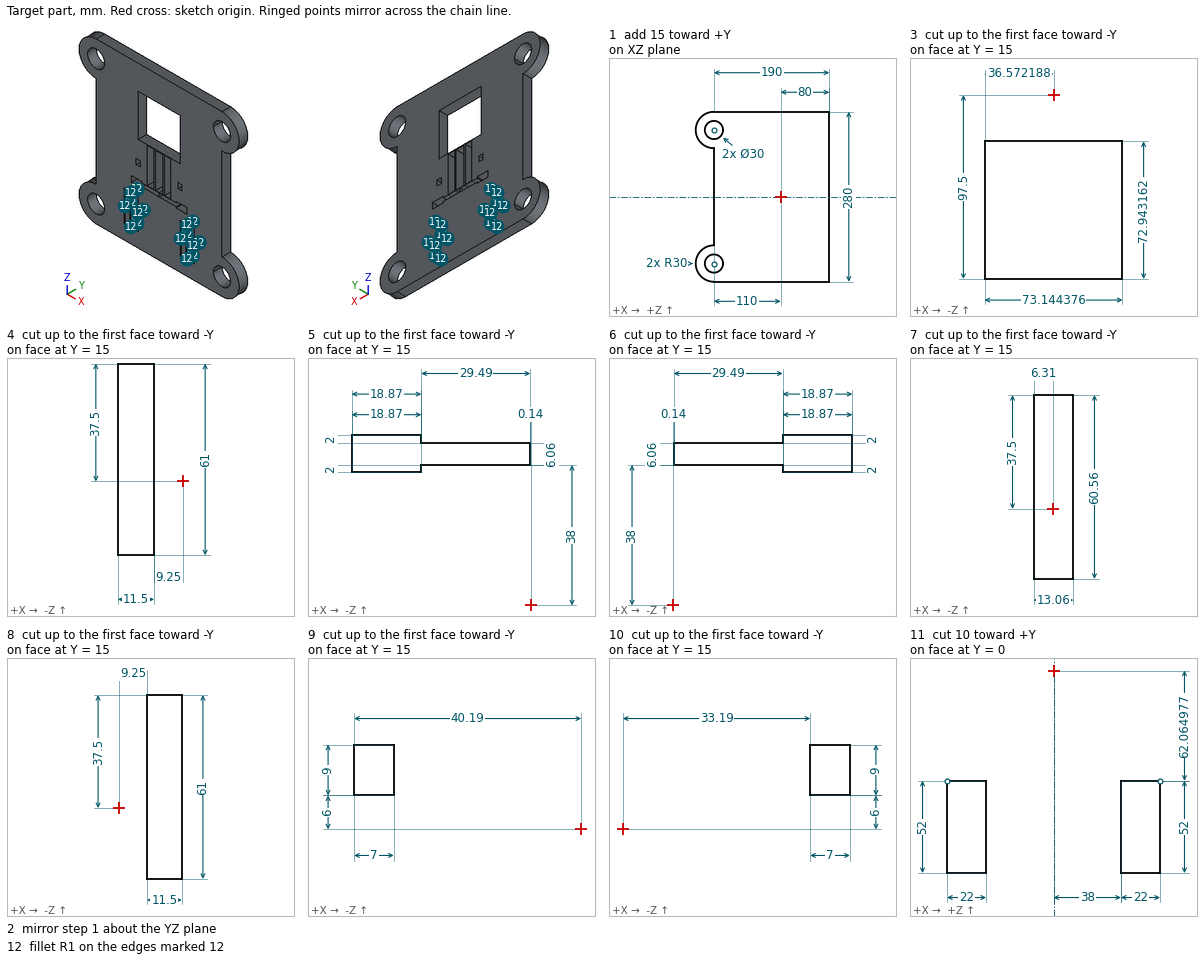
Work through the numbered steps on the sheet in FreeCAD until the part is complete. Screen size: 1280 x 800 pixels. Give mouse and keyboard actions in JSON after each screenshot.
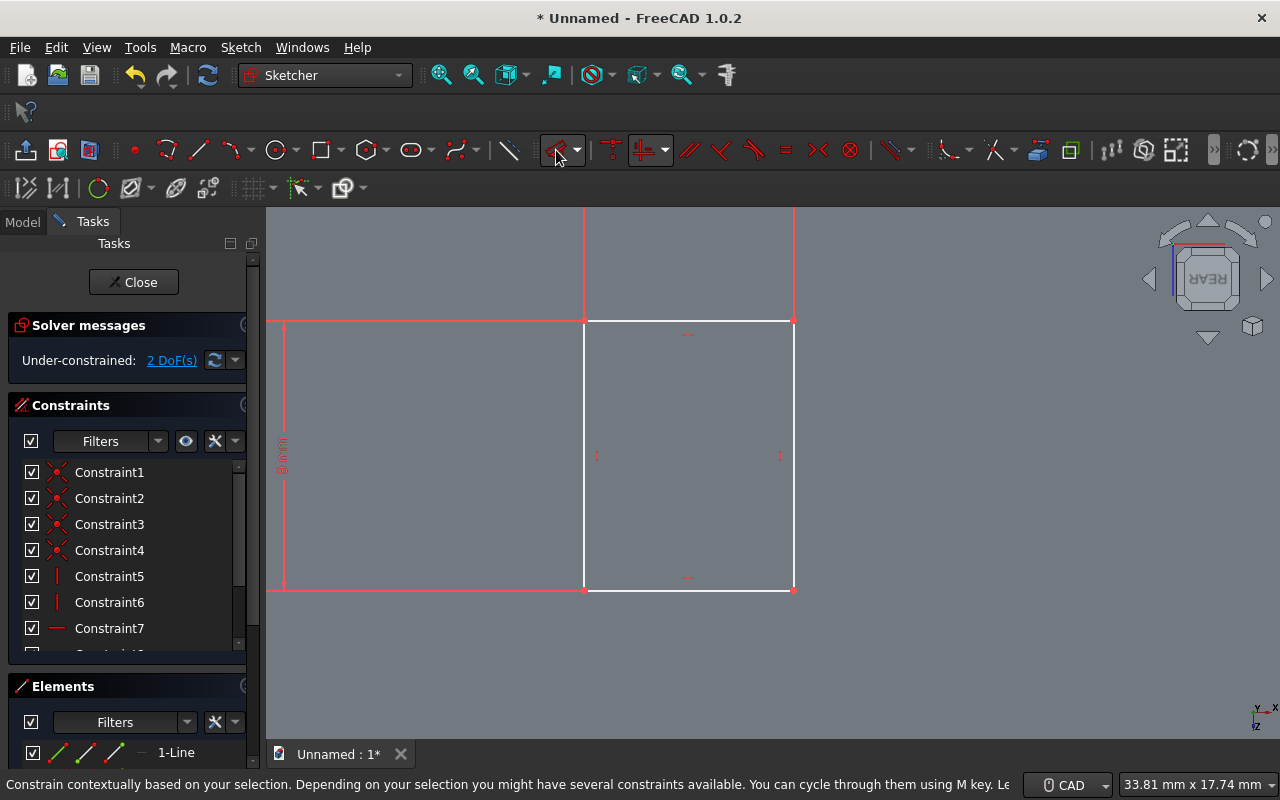
{"action": "left_click", "coordinate": [584, 591]}
{"action": "left_click", "coordinate": [618, 651]}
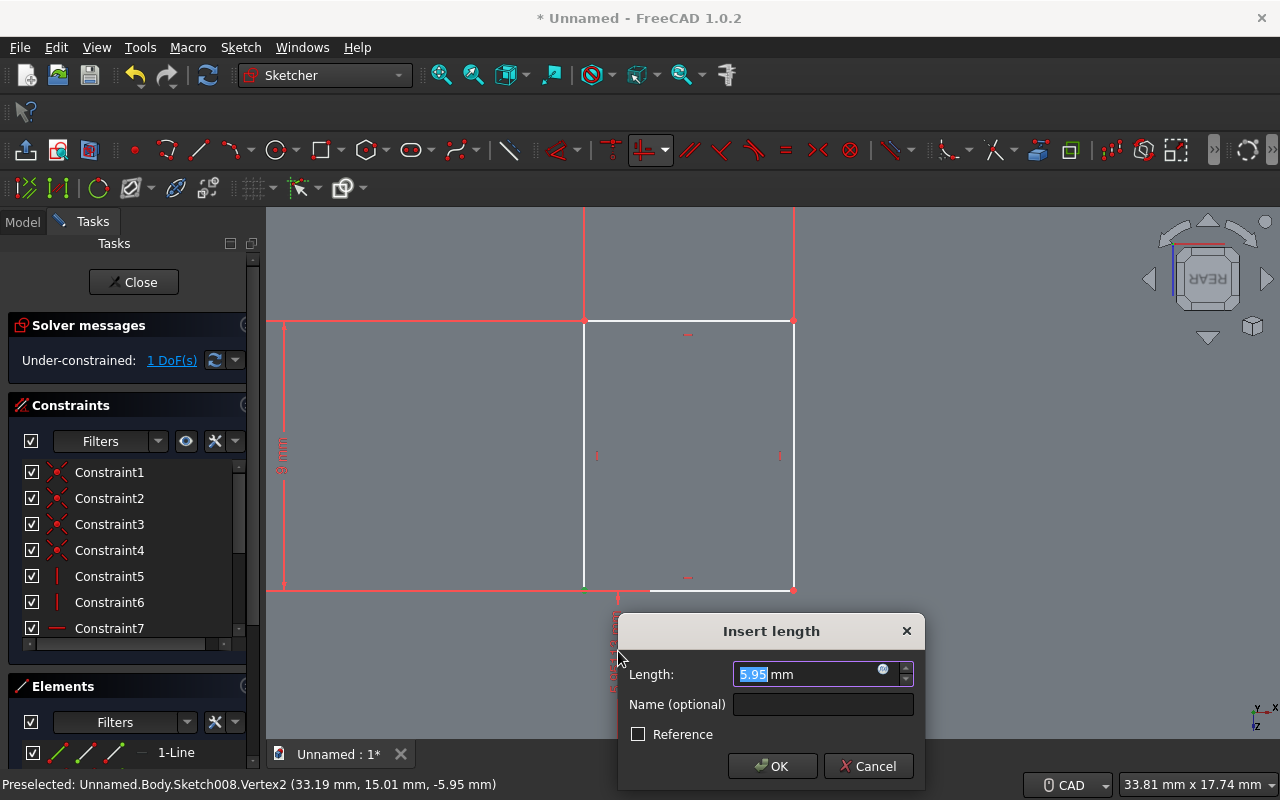
{"action": "type", "text": "6"}
{"action": "key", "text": "Return"}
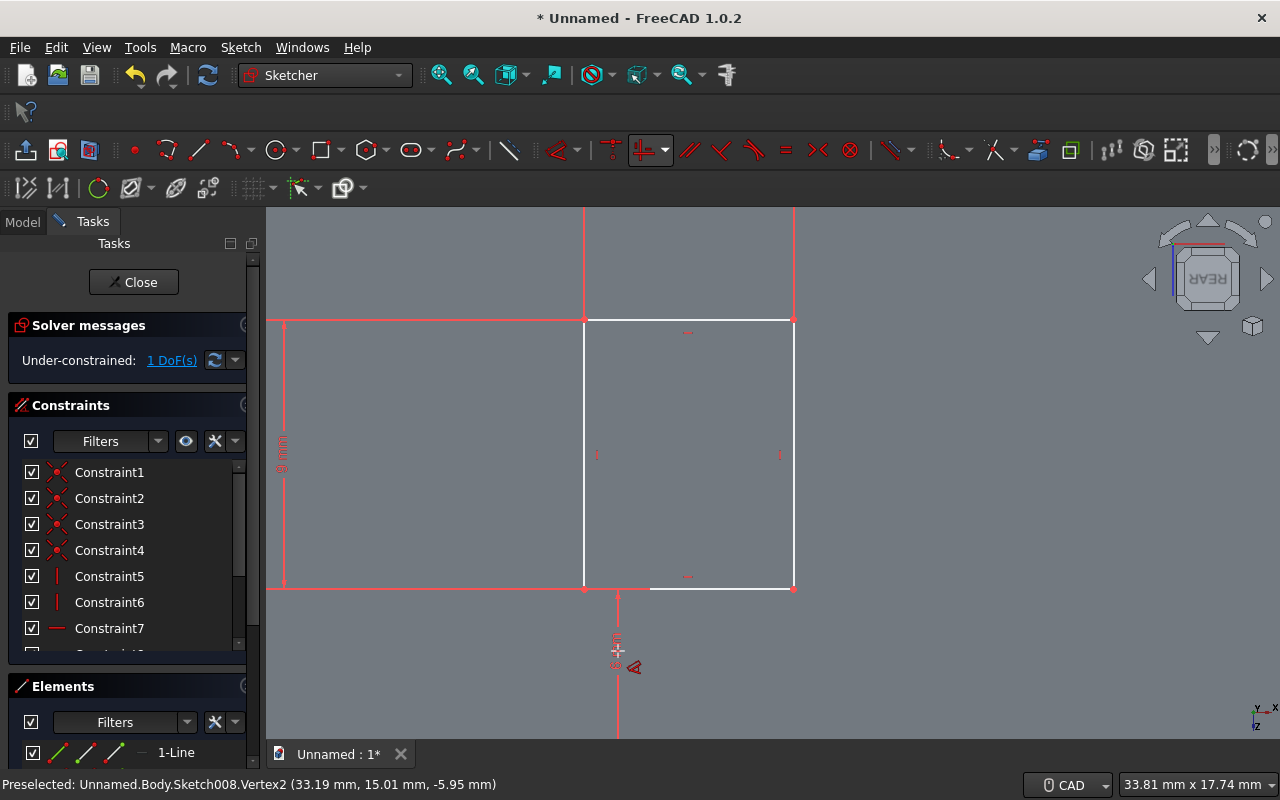
{"action": "left_click", "coordinate": [584, 320]}
{"action": "left_click", "coordinate": [439, 286]}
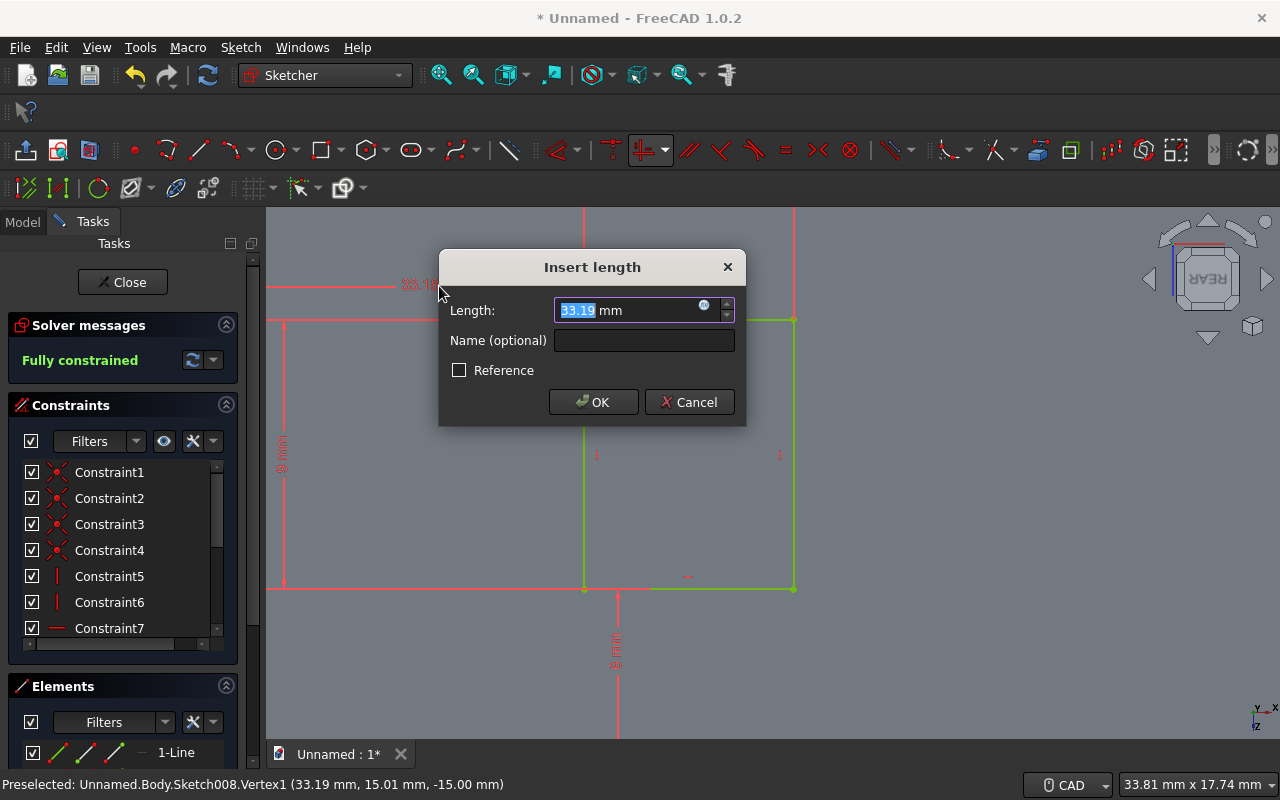
{"action": "type", "text": "33.19"}
{"action": "key", "text": "Return"}
{"action": "key", "text": "Escape"}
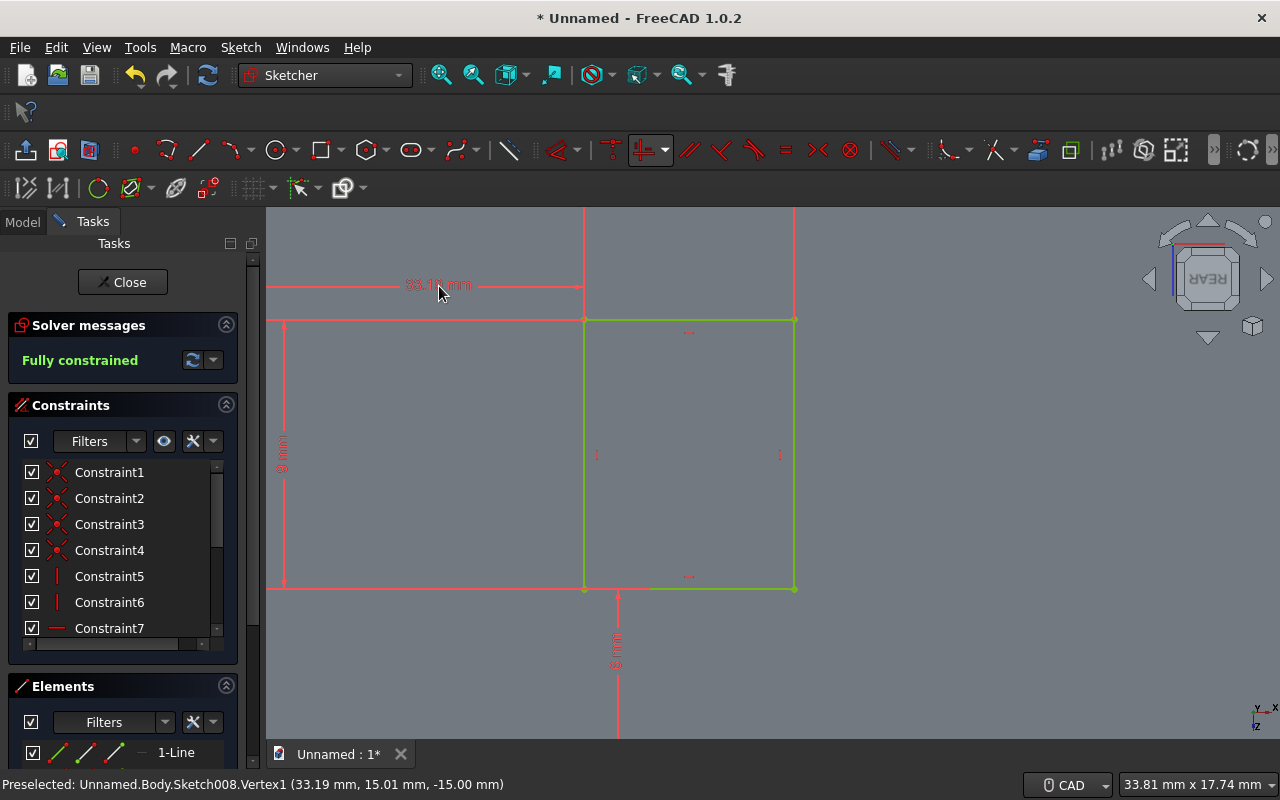
{"action": "left_click", "coordinate": [123, 282]}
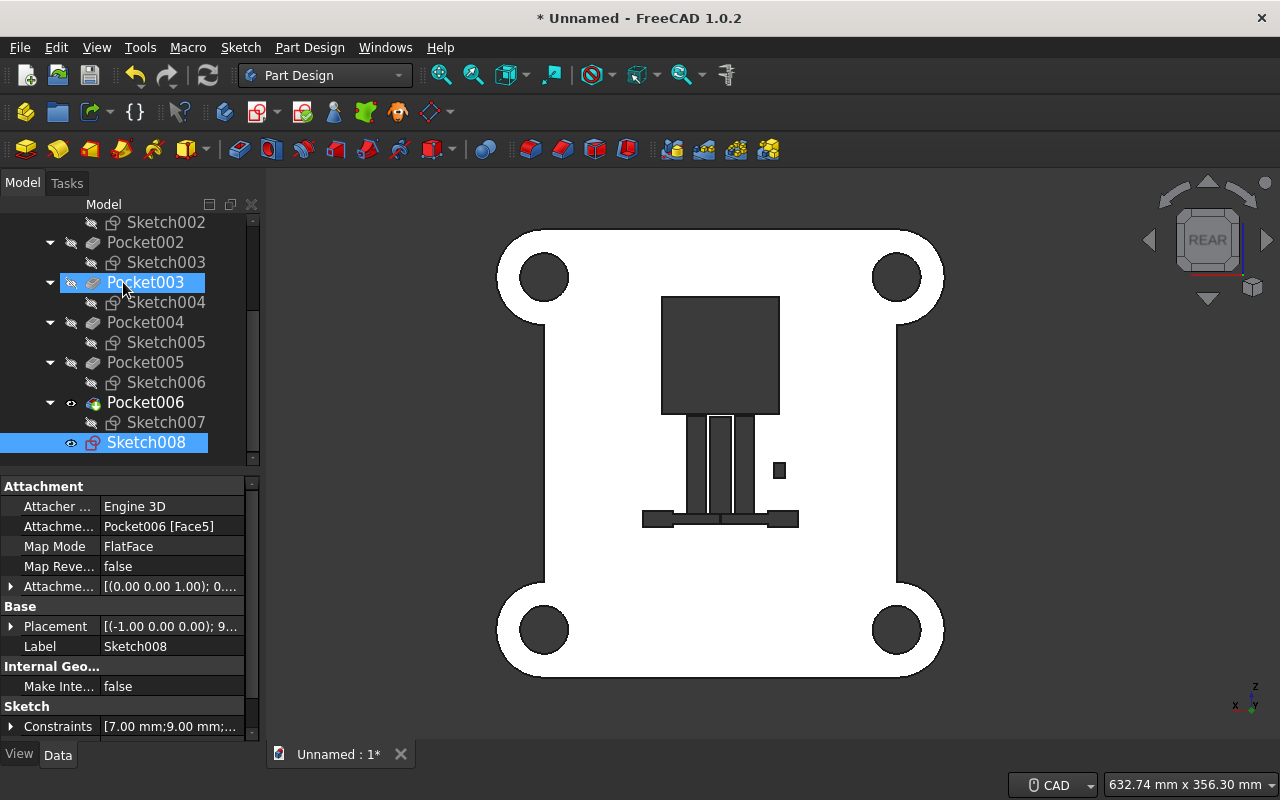
{"action": "left_click", "coordinate": [240, 150]}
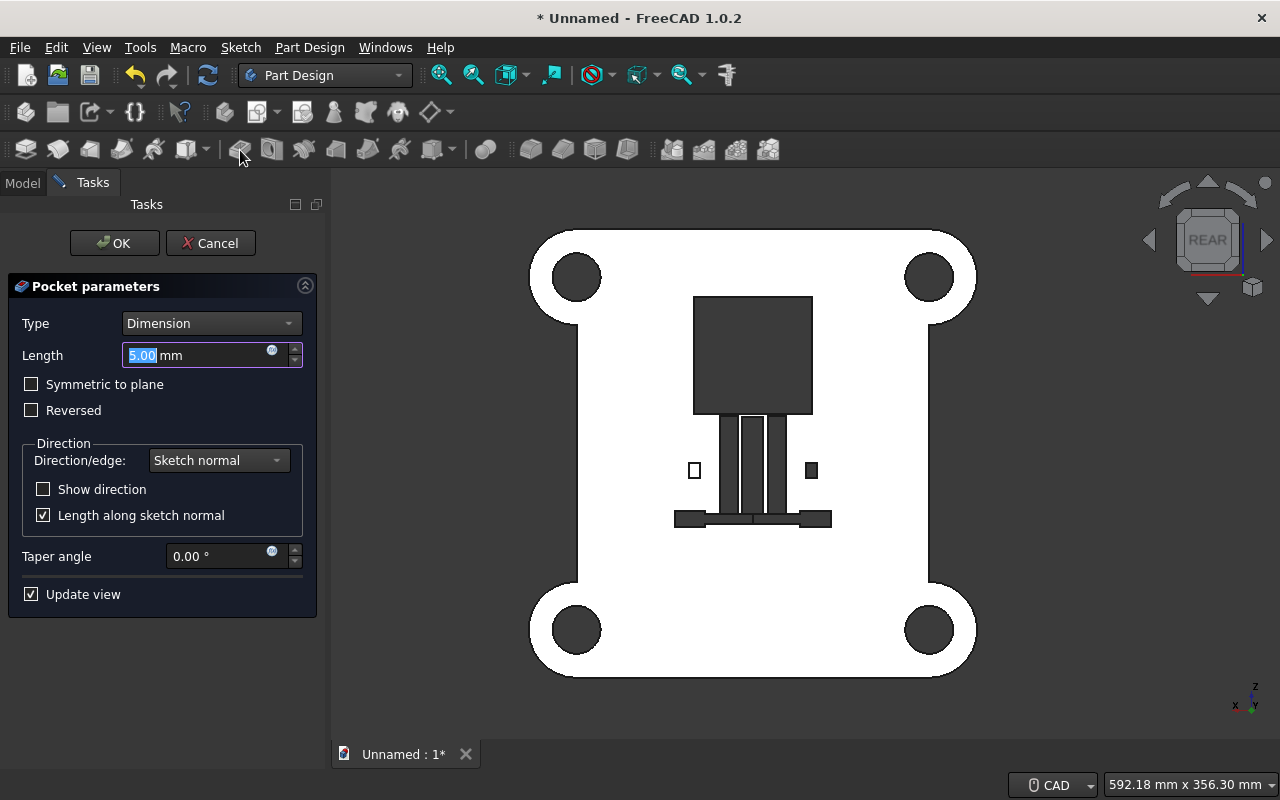
{"action": "left_click", "coordinate": [212, 324]}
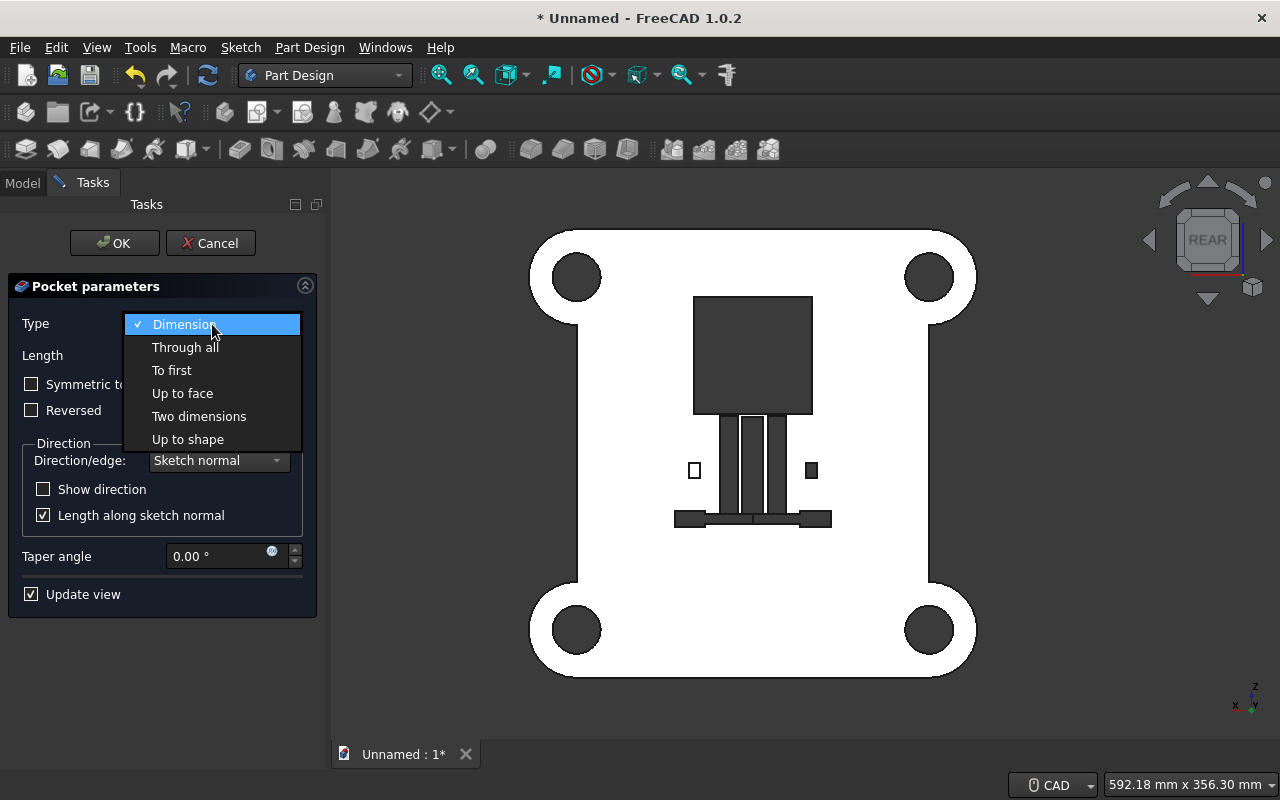
{"action": "left_click", "coordinate": [212, 370]}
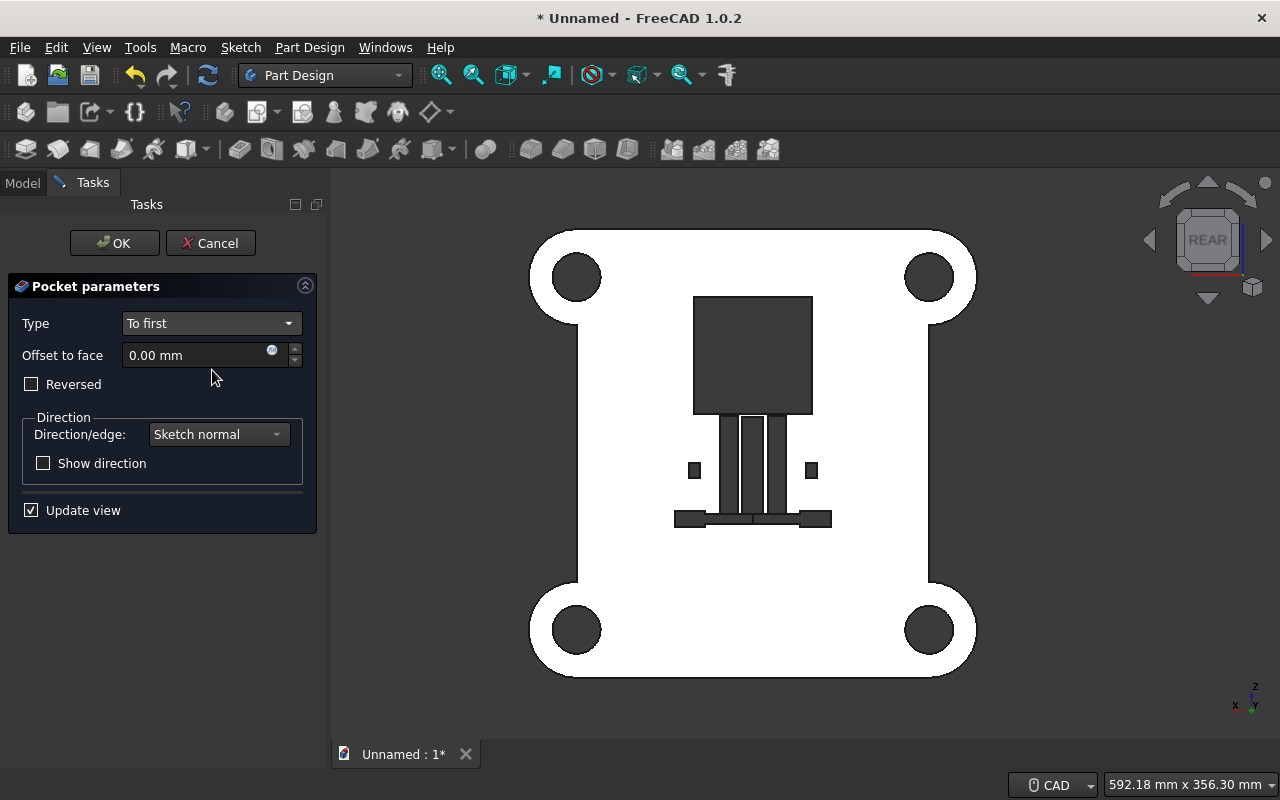
{"action": "left_click", "coordinate": [115, 243]}